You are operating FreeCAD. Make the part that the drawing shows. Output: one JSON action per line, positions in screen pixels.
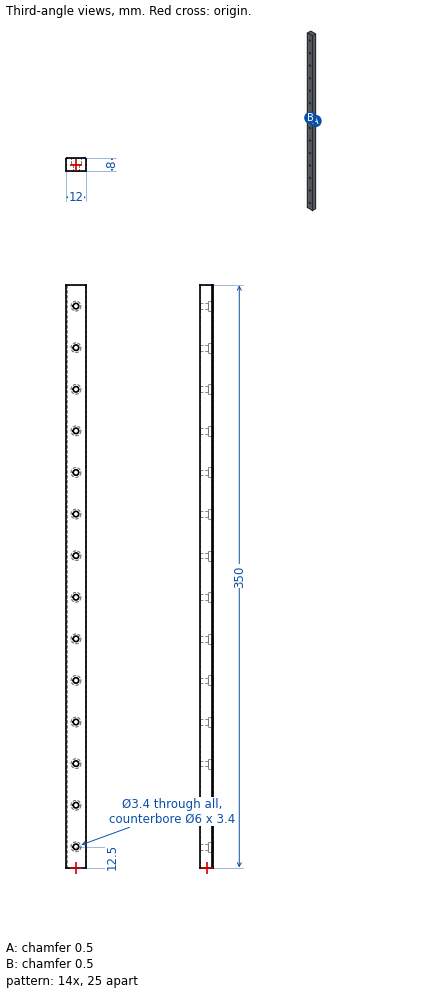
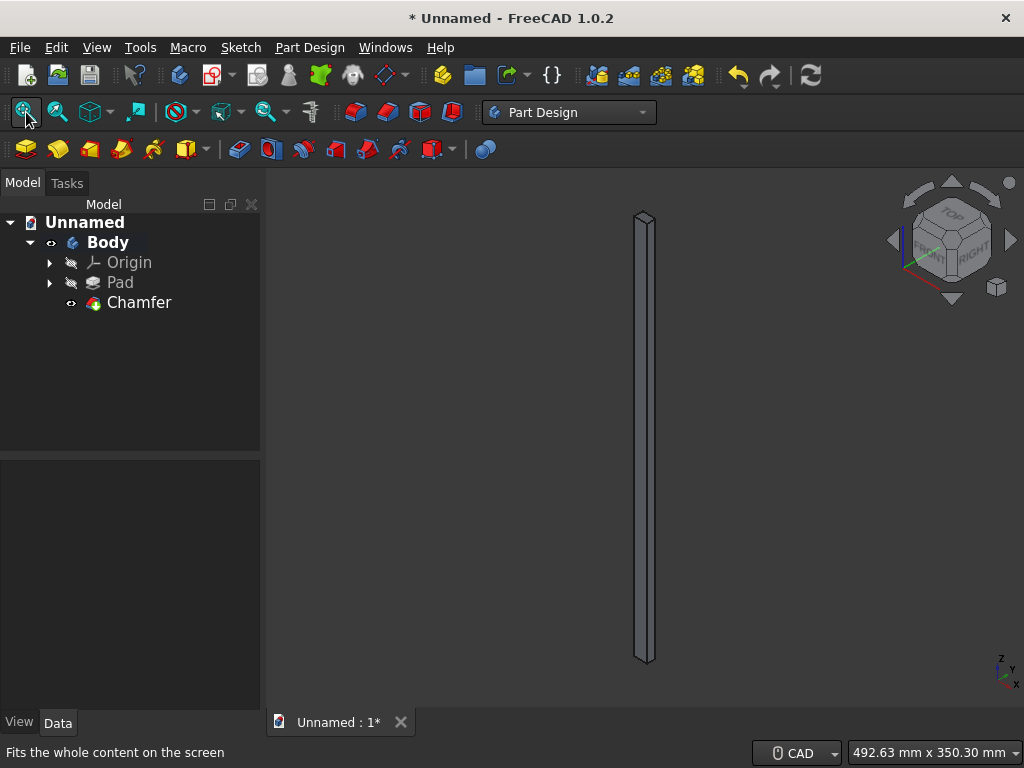
{"action": "key", "text": "2"}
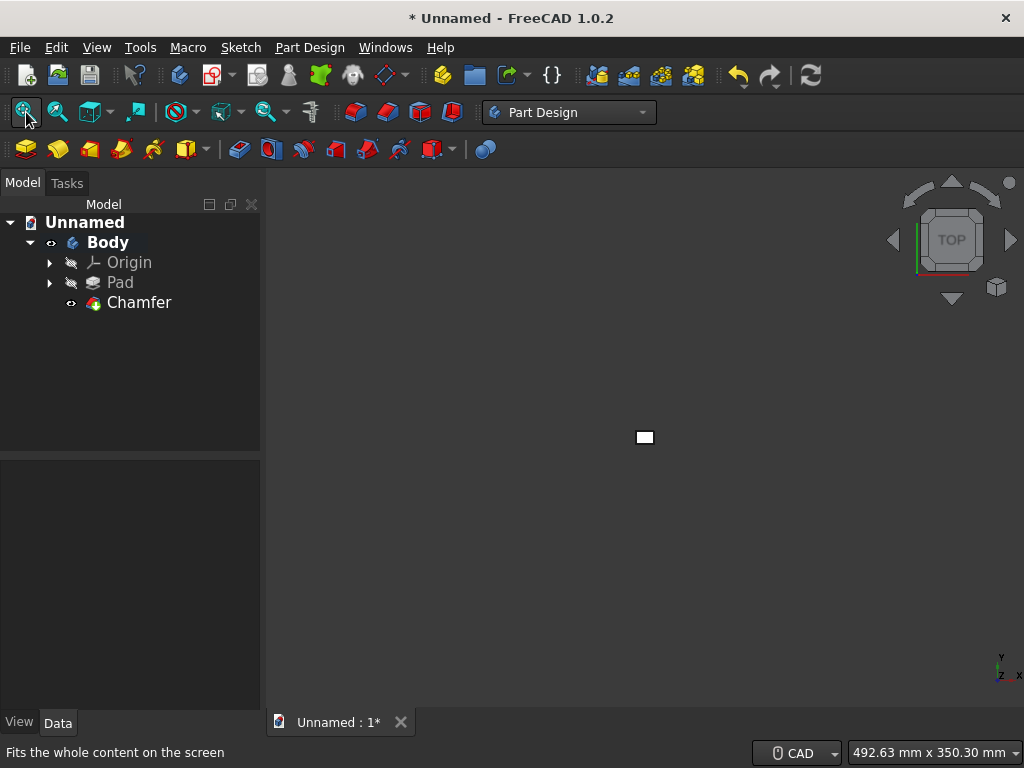
{"action": "left_click", "coordinate": [26, 112]}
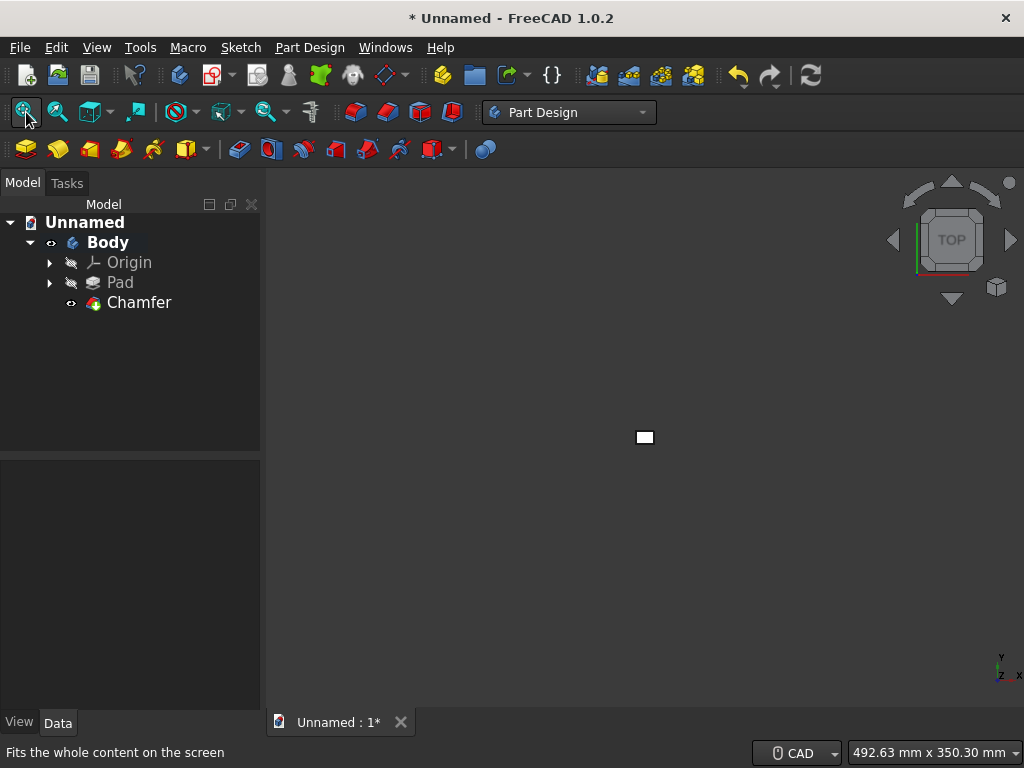
{"action": "key", "text": "1"}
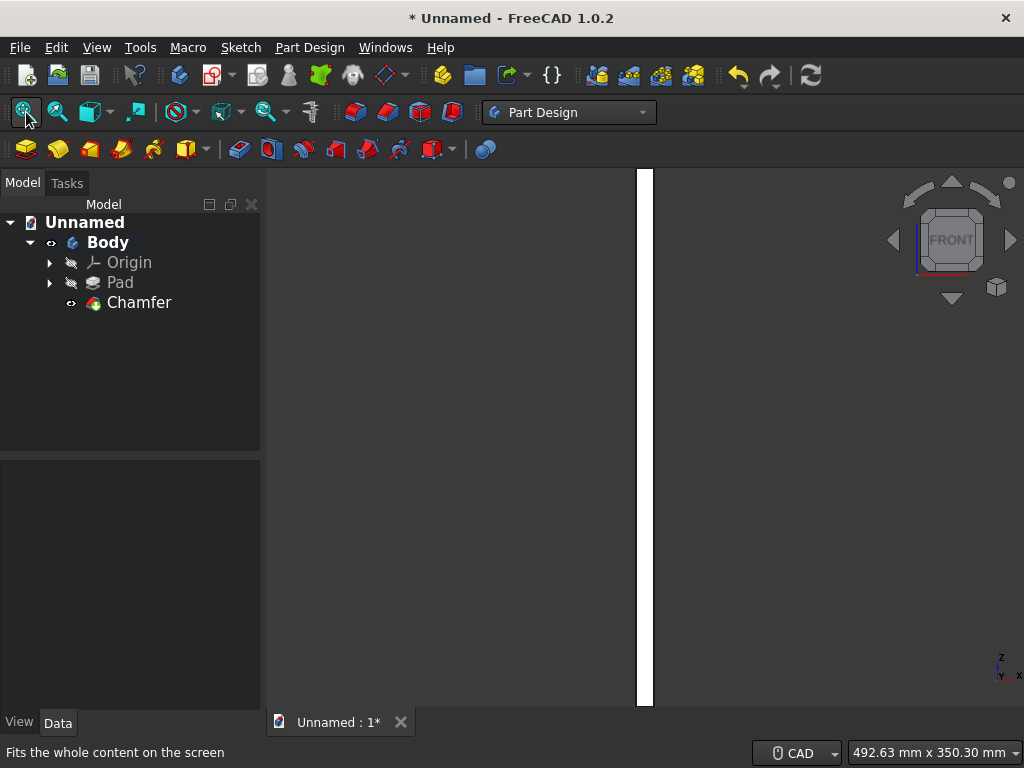
{"action": "left_click", "coordinate": [26, 112]}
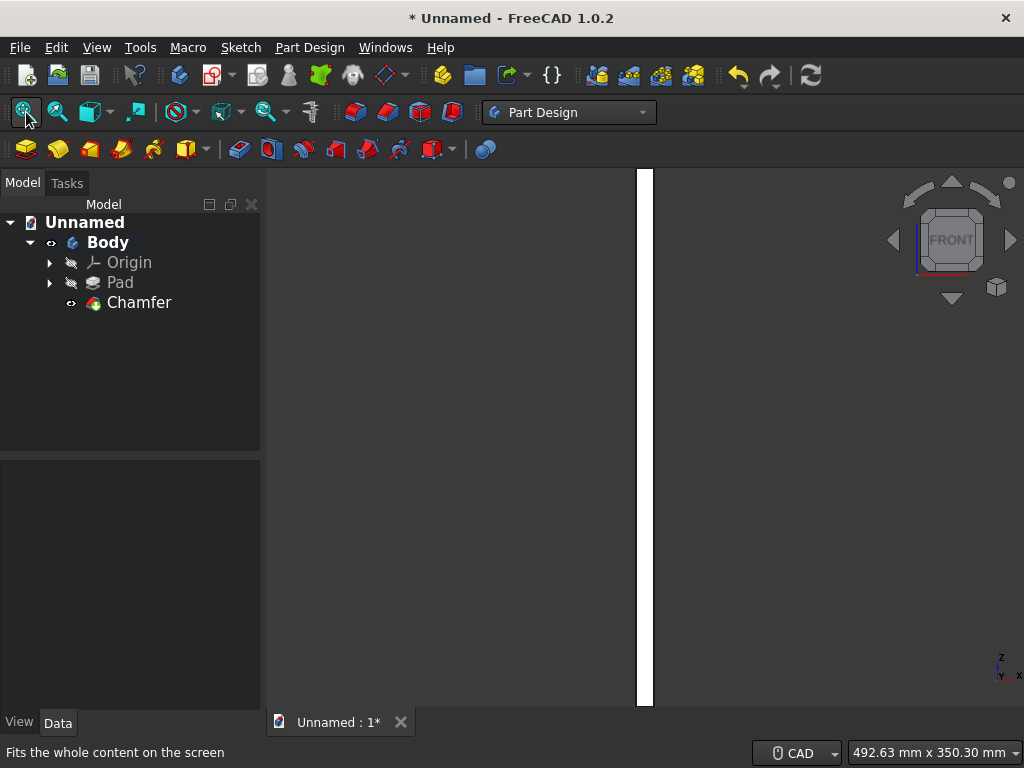
{"action": "key", "text": "3"}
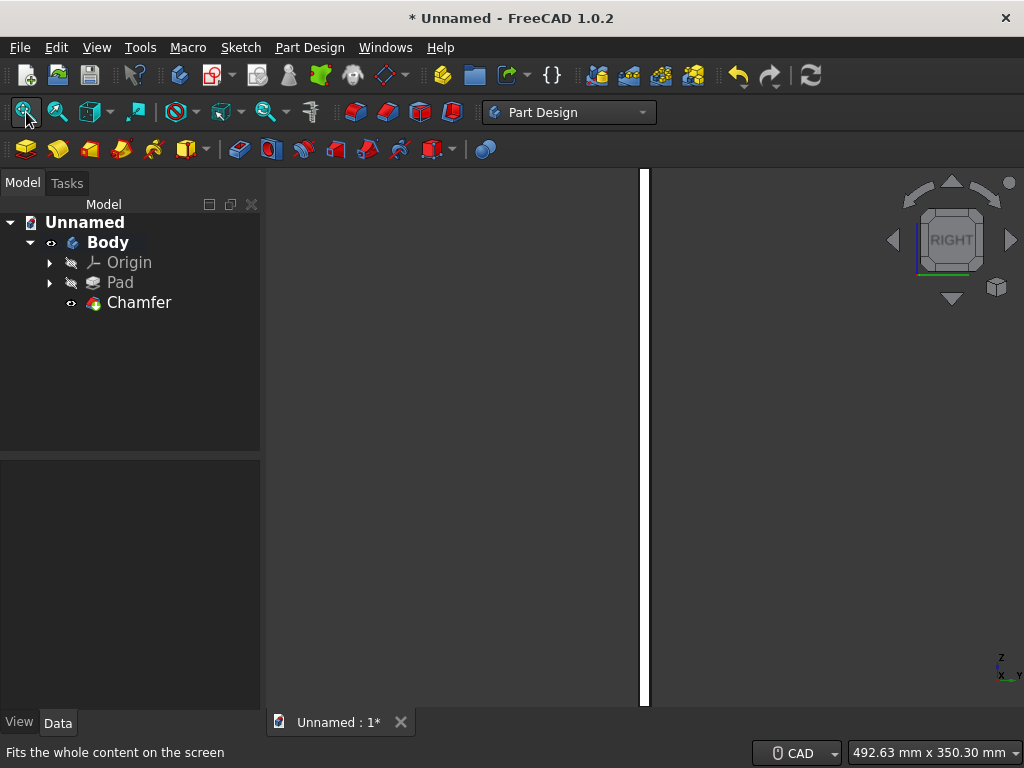
{"action": "left_click", "coordinate": [26, 112]}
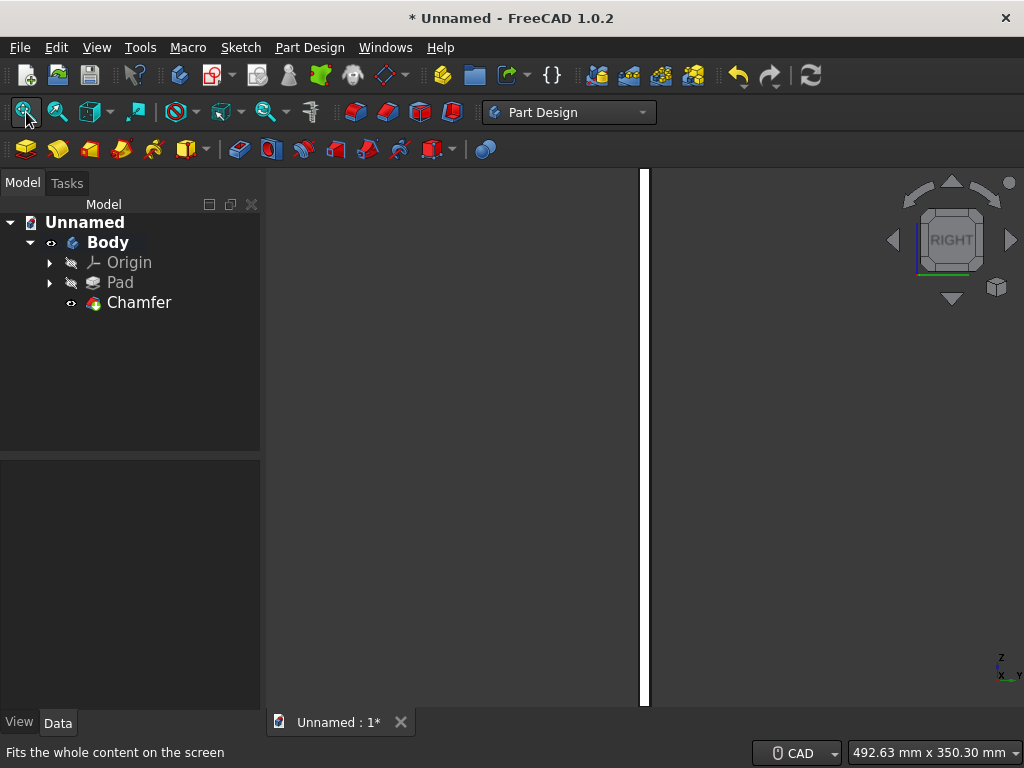
{"action": "key", "text": "5"}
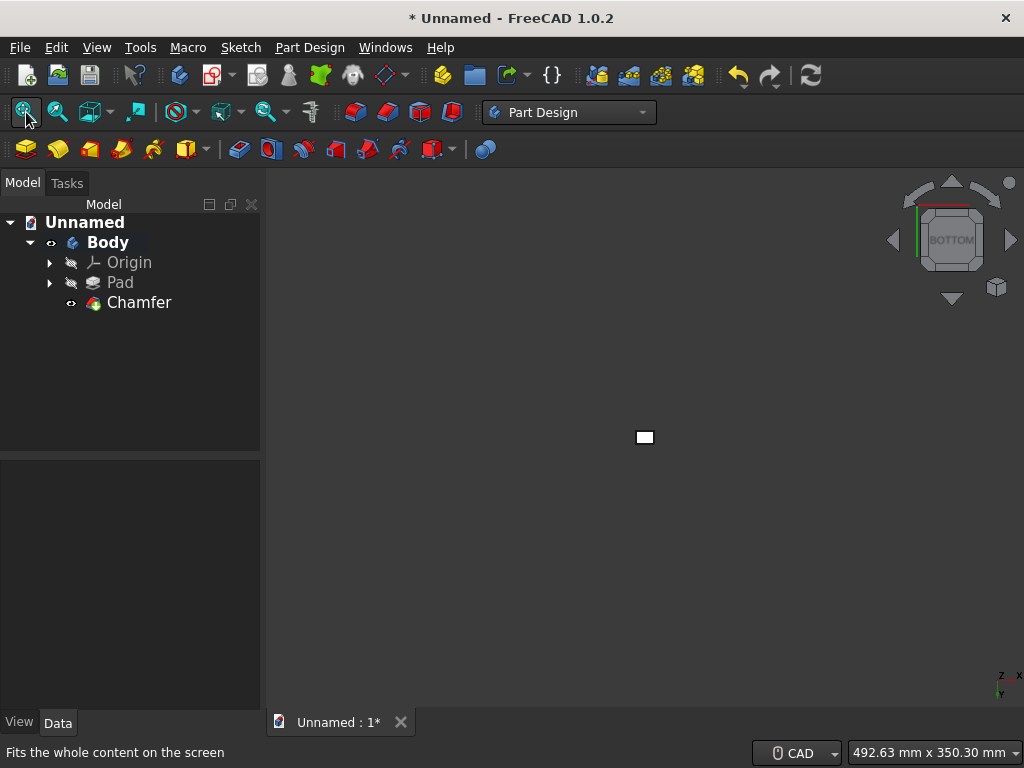
{"action": "left_click", "coordinate": [26, 112]}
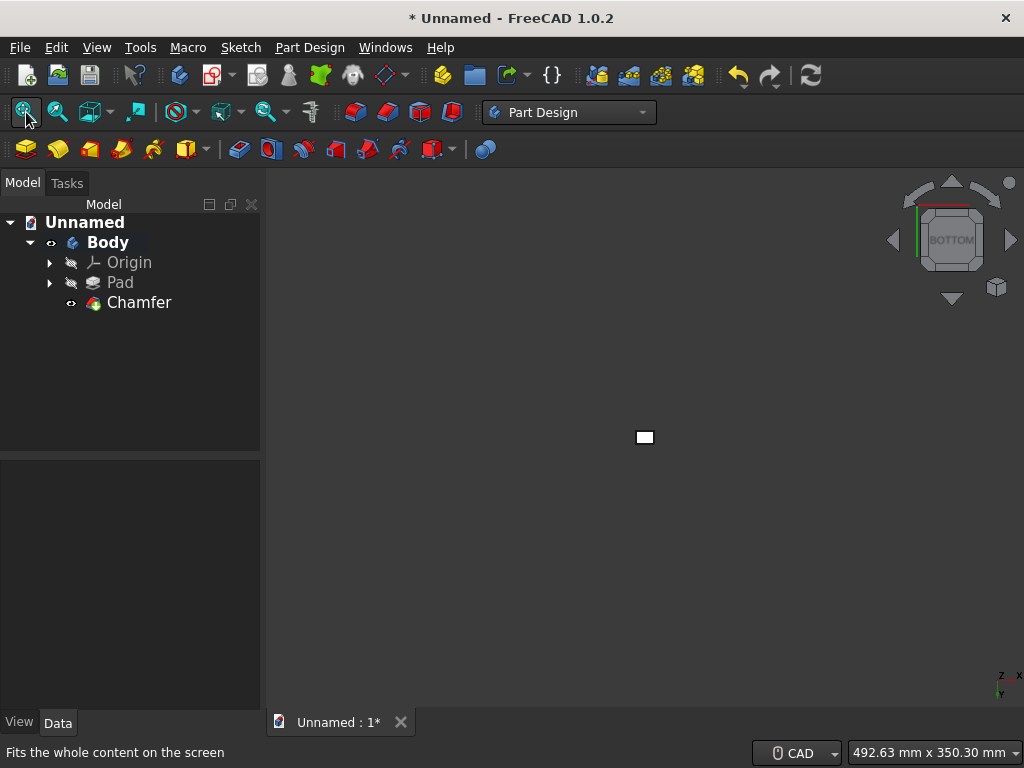
{"action": "key", "text": "4"}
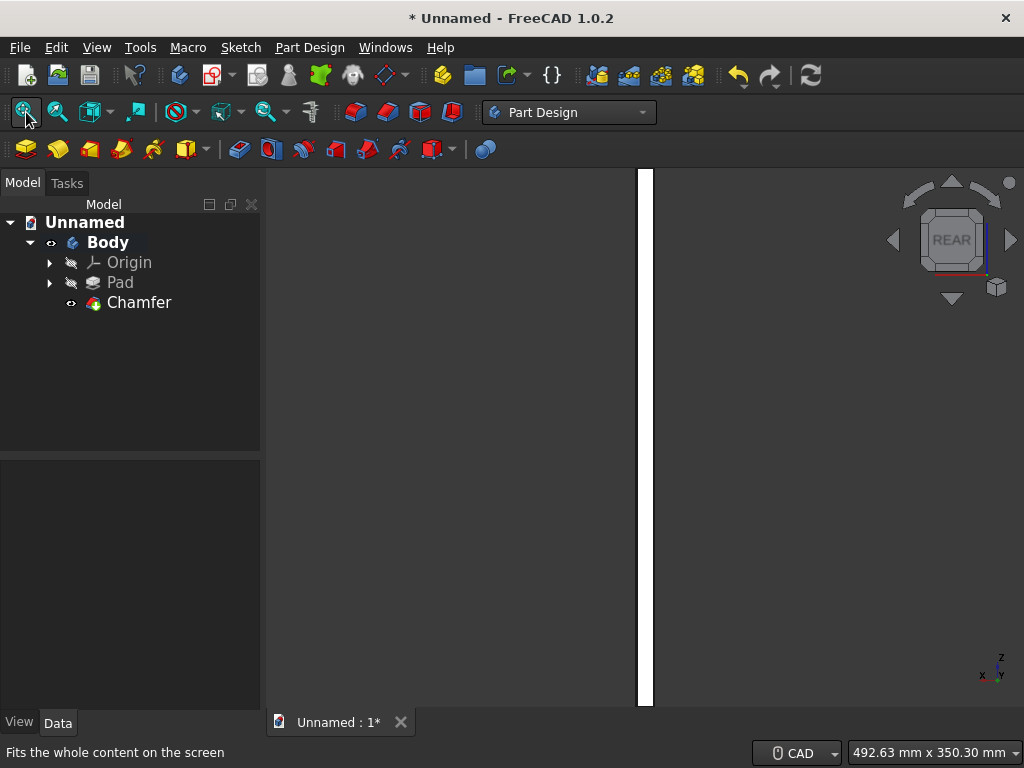
{"action": "left_click", "coordinate": [26, 112]}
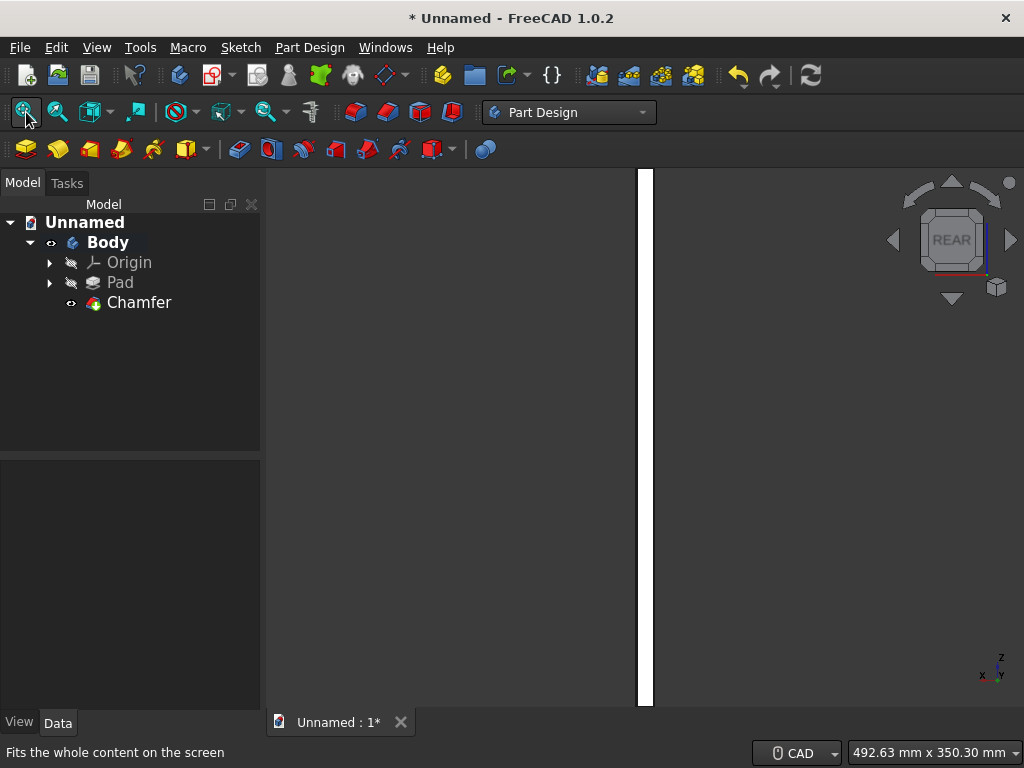
{"action": "left_click", "coordinate": [654, 437]}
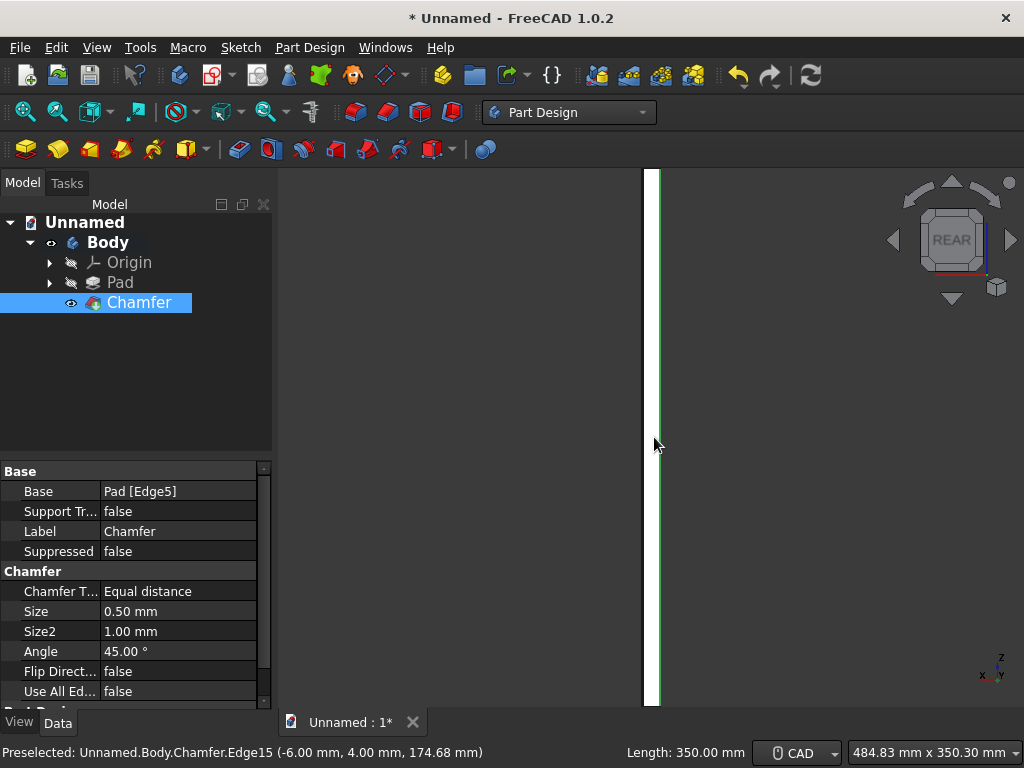
{"action": "left_click", "coordinate": [388, 112]}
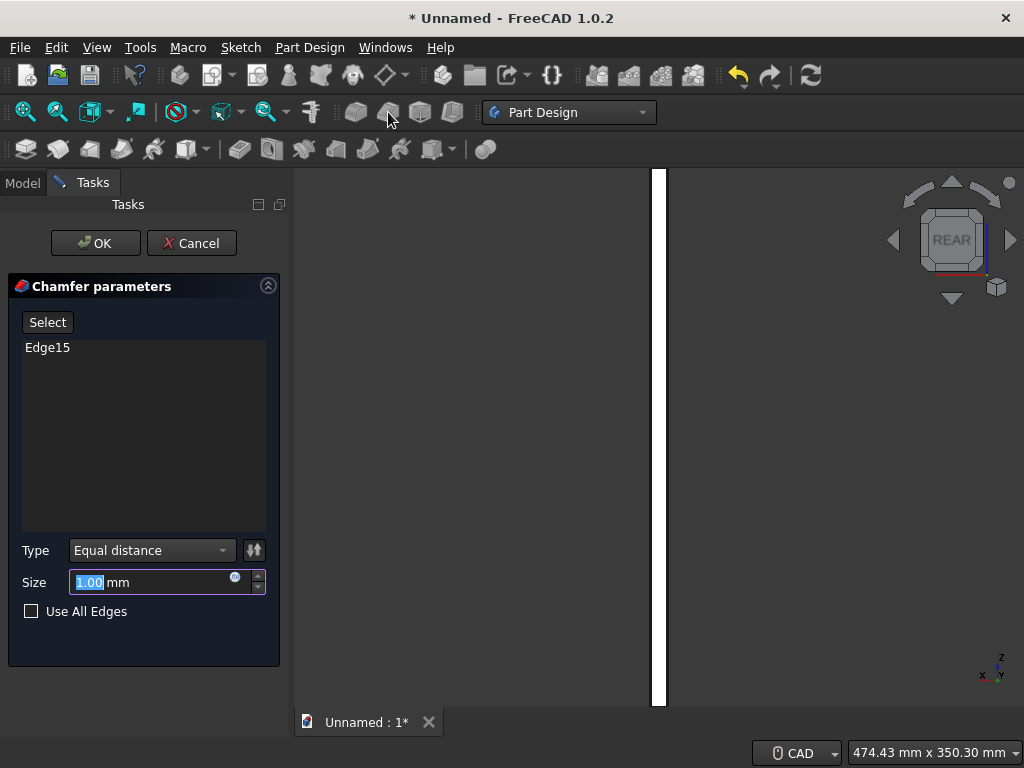
{"action": "type", "text": "0.5"}
{"action": "key", "text": "Tab"}